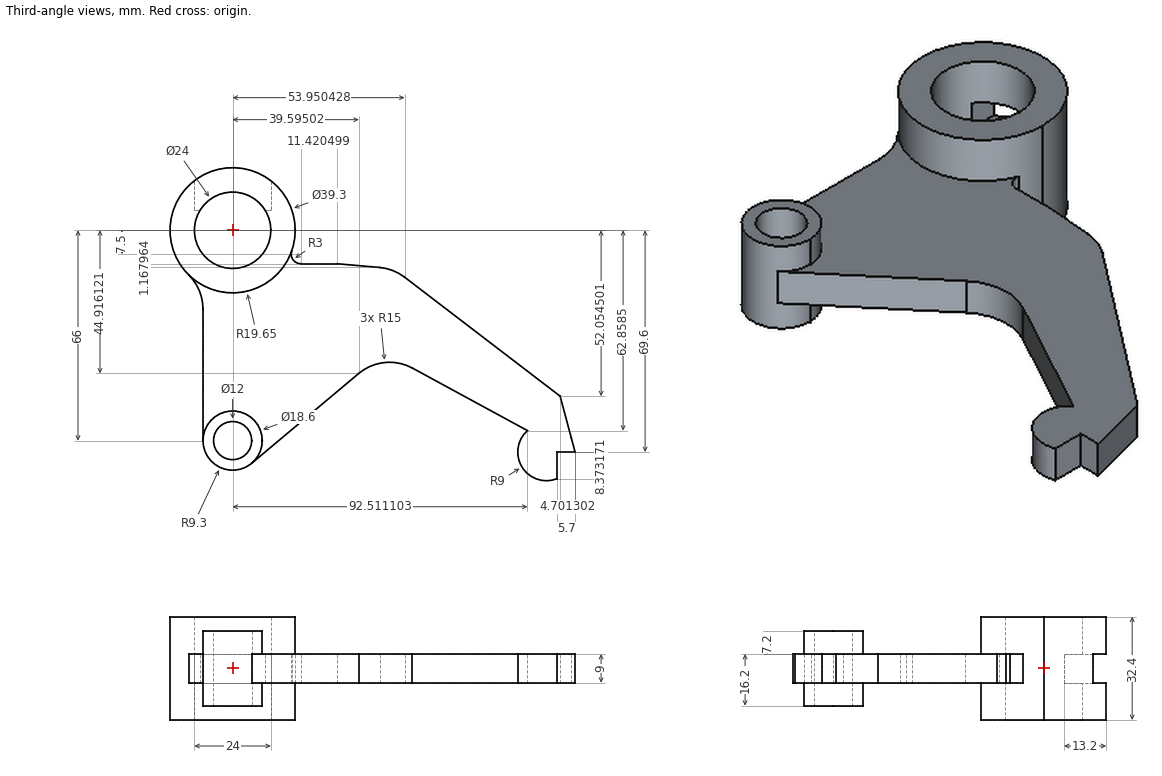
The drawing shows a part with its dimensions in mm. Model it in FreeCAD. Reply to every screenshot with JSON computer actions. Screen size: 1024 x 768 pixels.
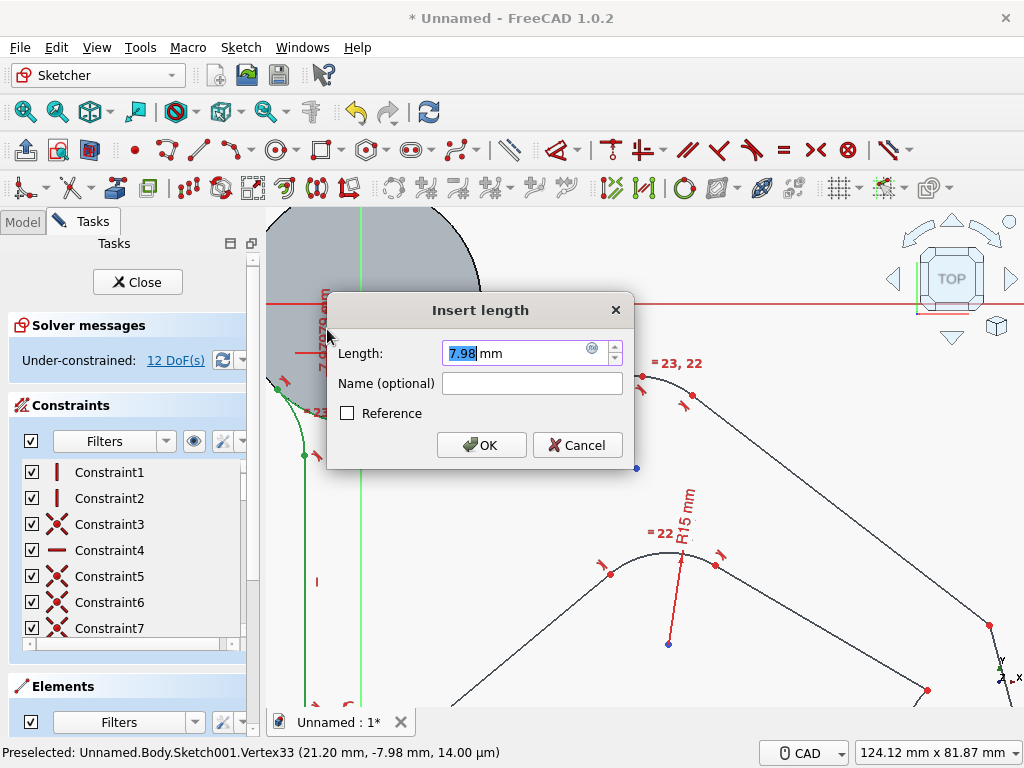
{"action": "type", "text": "7.5"}
{"action": "key", "text": "Return"}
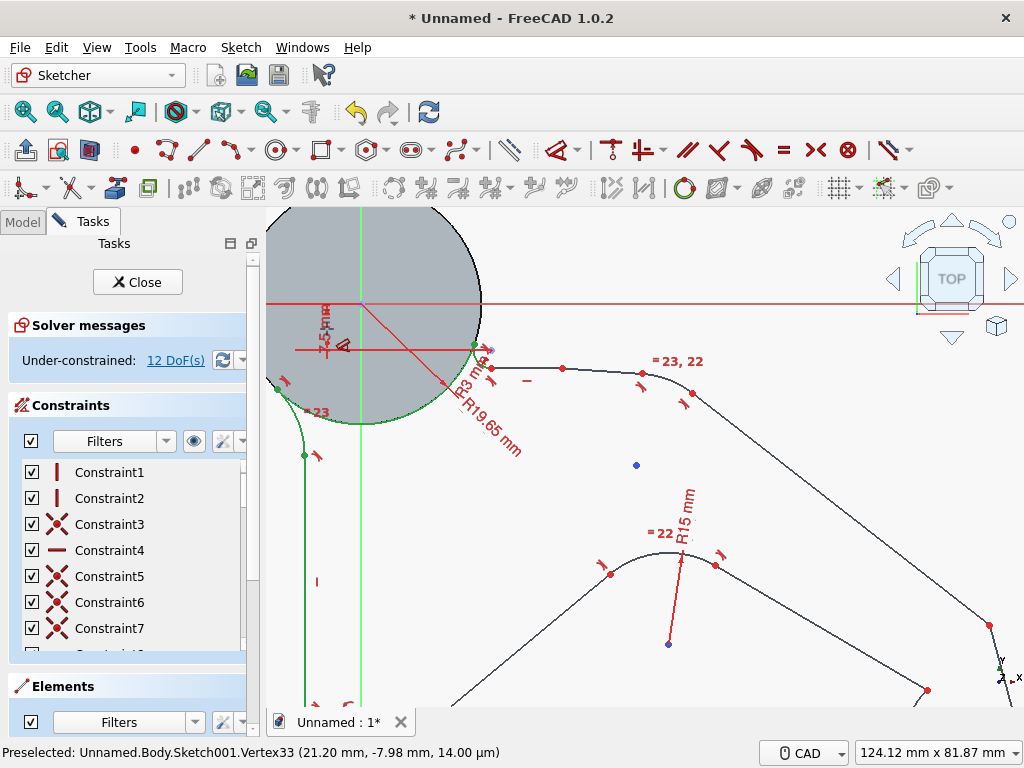
{"action": "scroll", "coordinate": [490, 353], "scroll_direction": "down", "scroll_amount": 3}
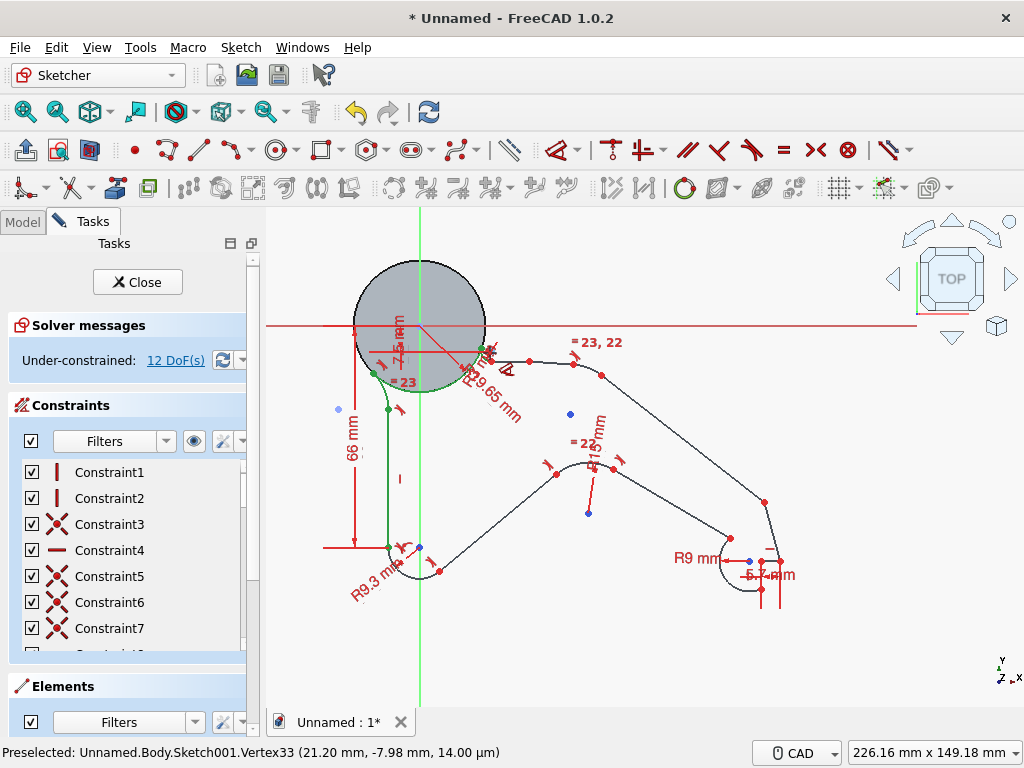
{"action": "left_click", "coordinate": [761, 561]}
{"action": "left_click", "coordinate": [795, 444]}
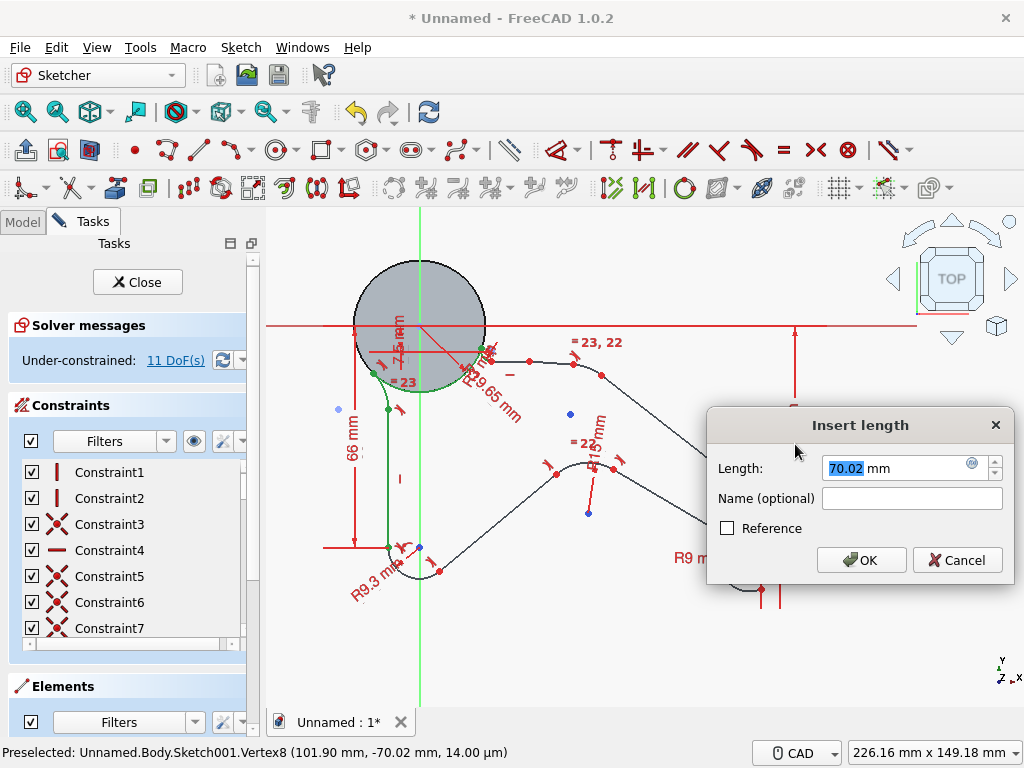
{"action": "type", "text": "69.6"}
{"action": "key", "text": "Return"}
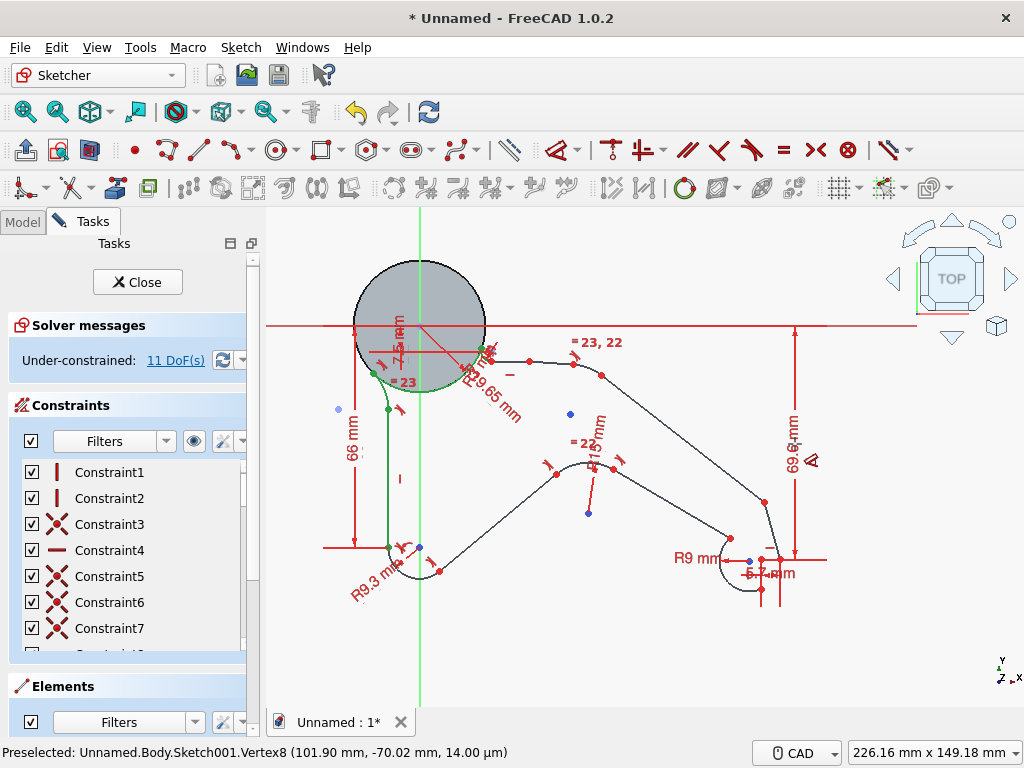
{"action": "left_click", "coordinate": [750, 561]}
{"action": "left_click", "coordinate": [784, 390]}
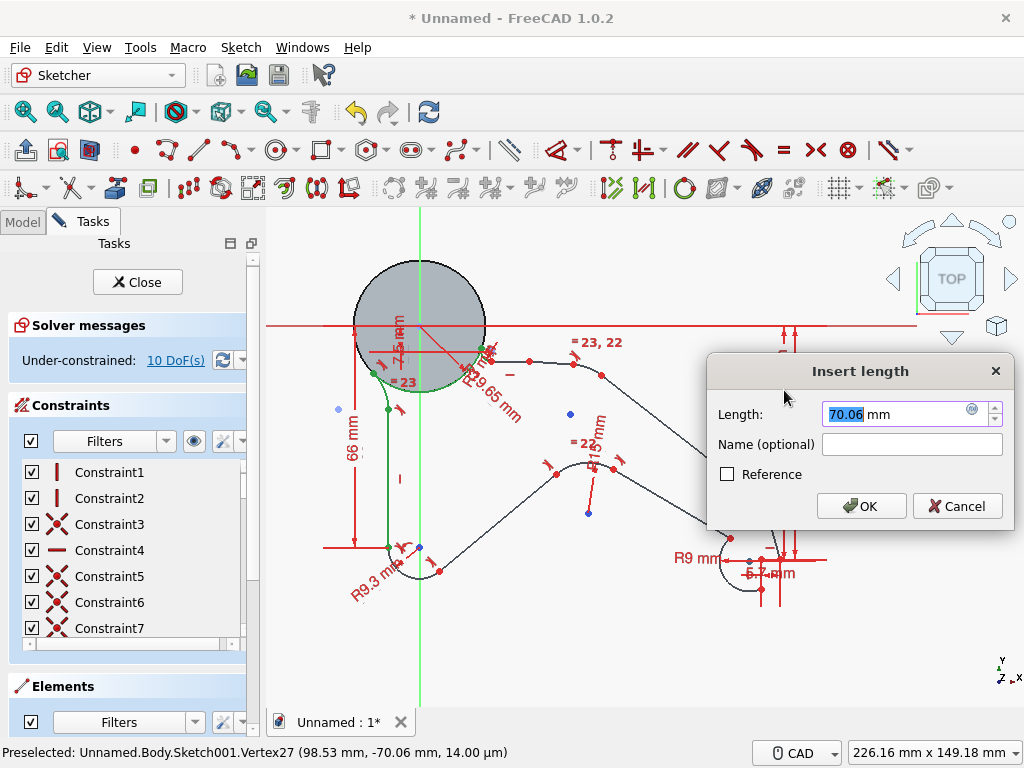
{"action": "type", "text": "69.6"}
{"action": "key", "text": "Return"}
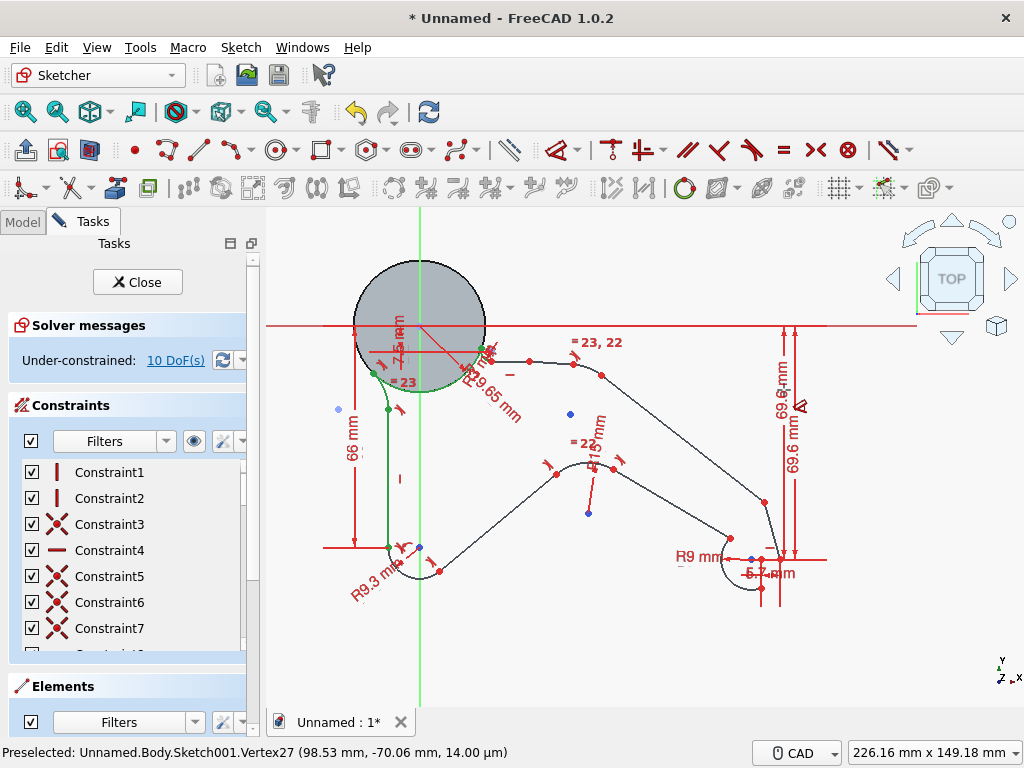
{"action": "scroll", "coordinate": [761, 577], "scroll_direction": "up", "scroll_amount": 2}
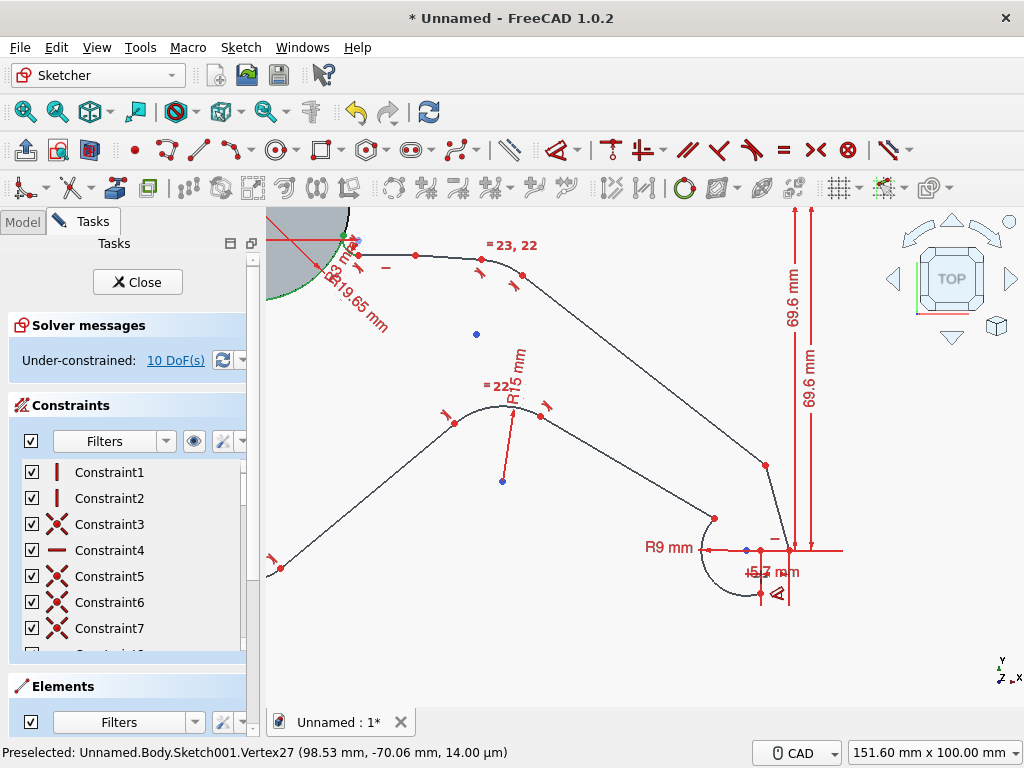
{"action": "left_click", "coordinate": [761, 576]}
{"action": "left_click", "coordinate": [679, 572]}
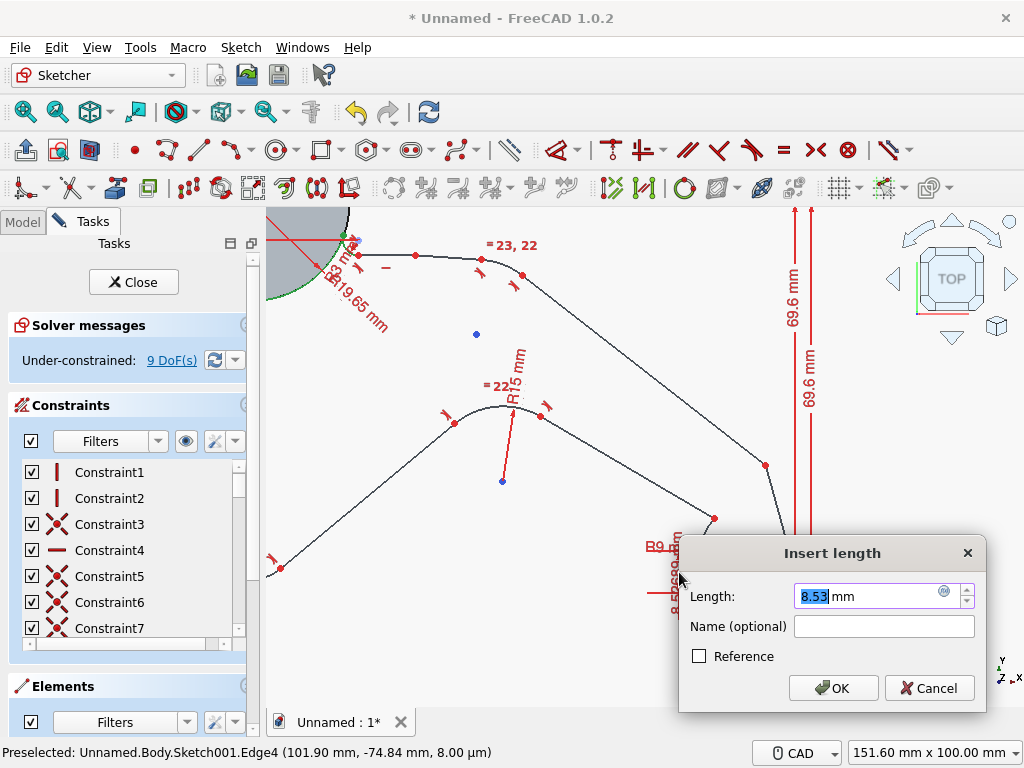
{"action": "type", "text": "8.373171"}
{"action": "key", "text": "Return"}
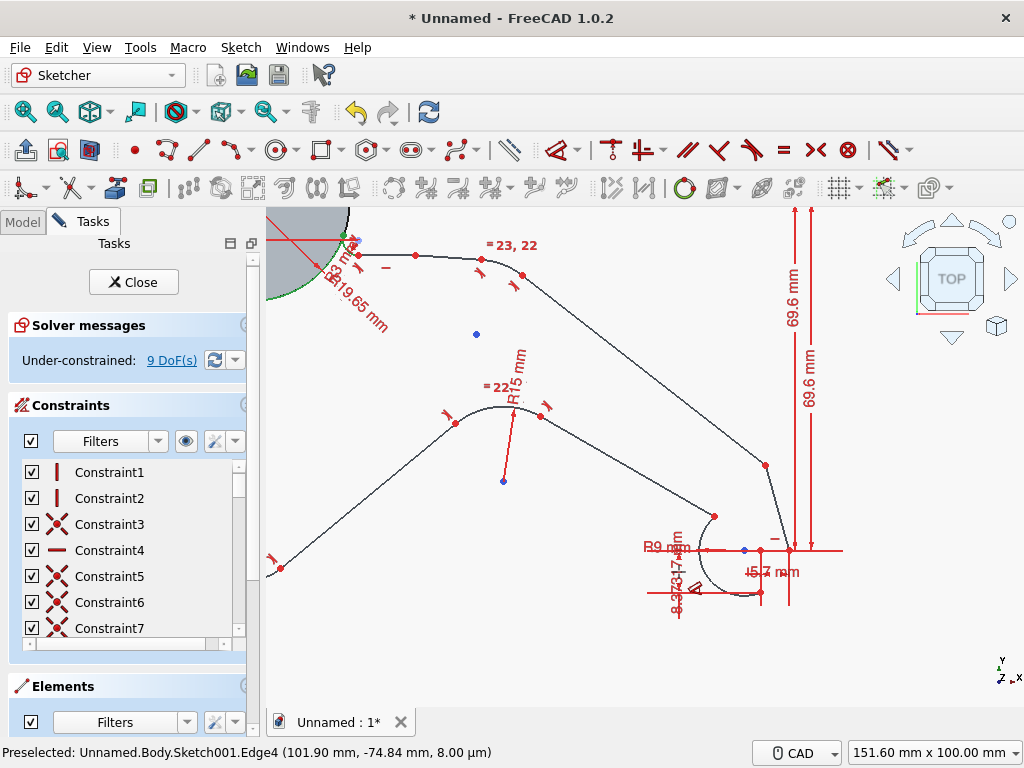
{"action": "left_click", "coordinate": [715, 517]}
{"action": "left_click", "coordinate": [749, 277]}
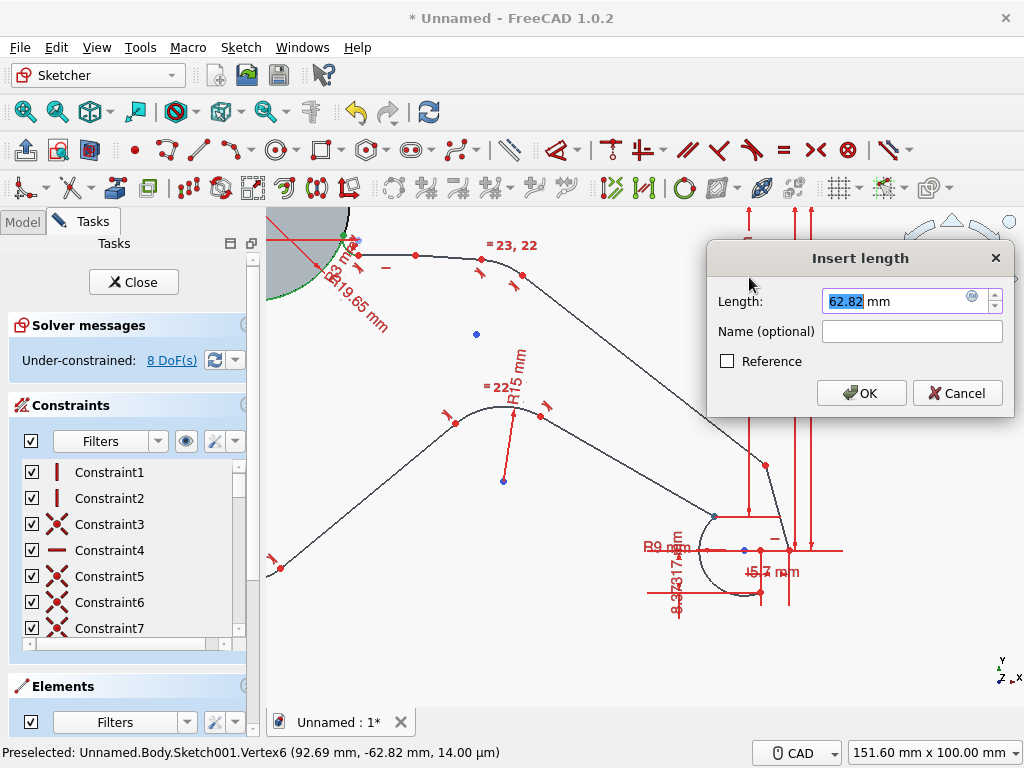
{"action": "type", "text": "62.8585"}
{"action": "key", "text": "Return"}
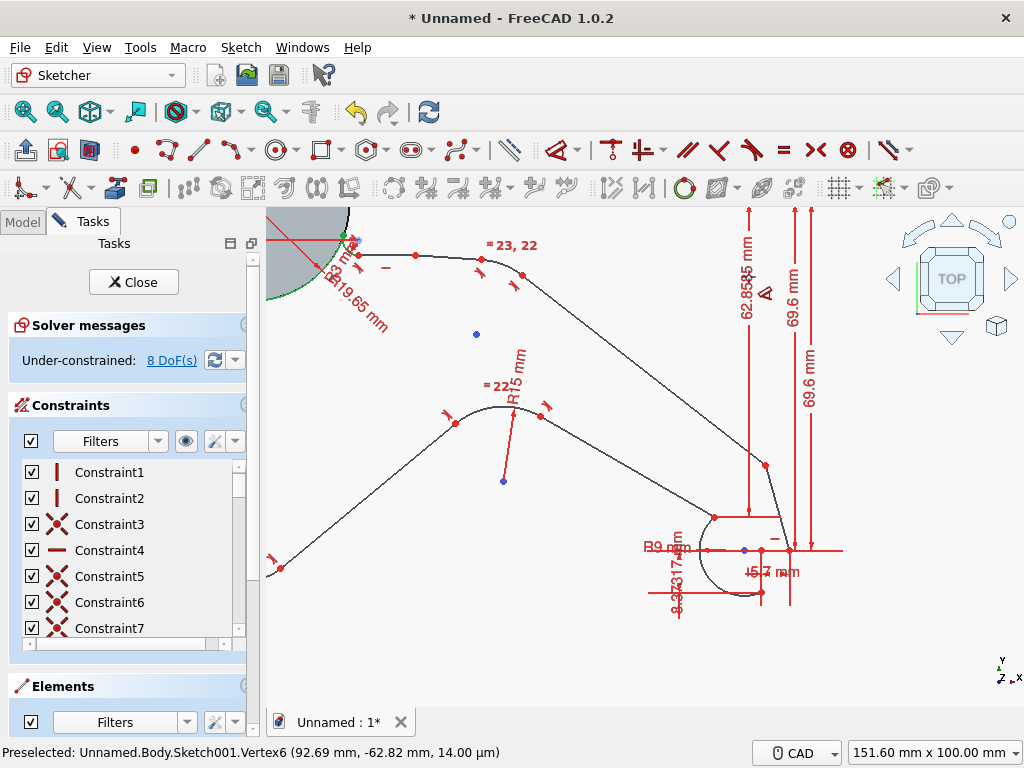
{"action": "left_click", "coordinate": [399, 255]}
{"action": "left_click", "coordinate": [387, 337]}